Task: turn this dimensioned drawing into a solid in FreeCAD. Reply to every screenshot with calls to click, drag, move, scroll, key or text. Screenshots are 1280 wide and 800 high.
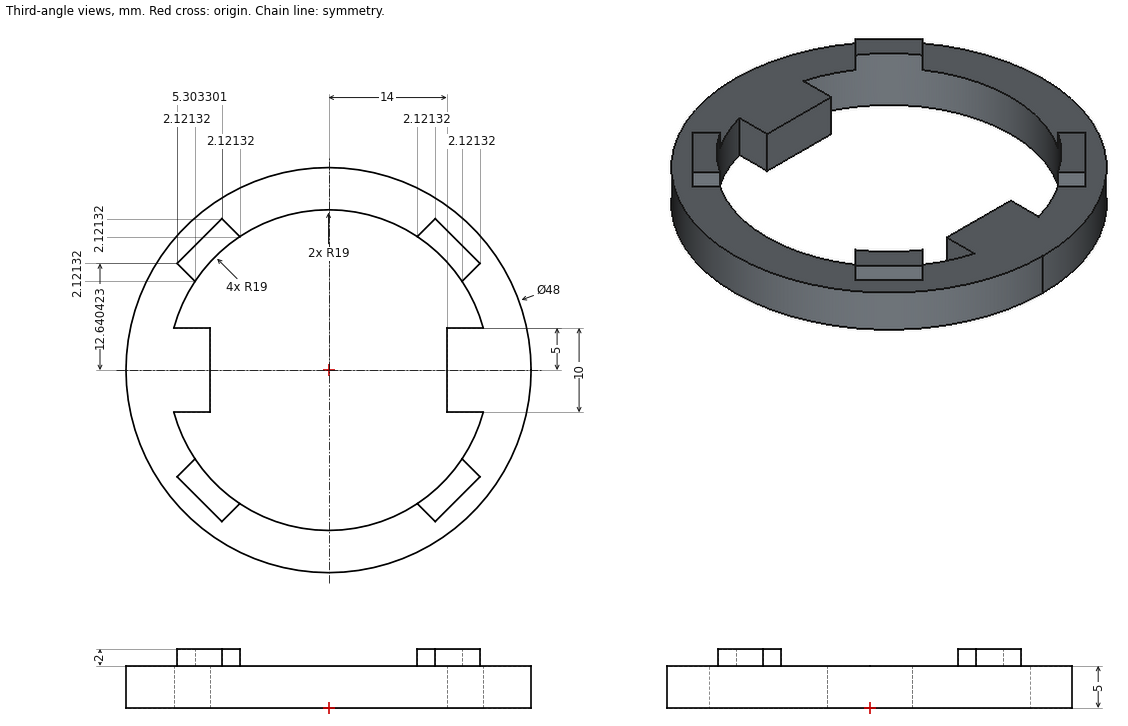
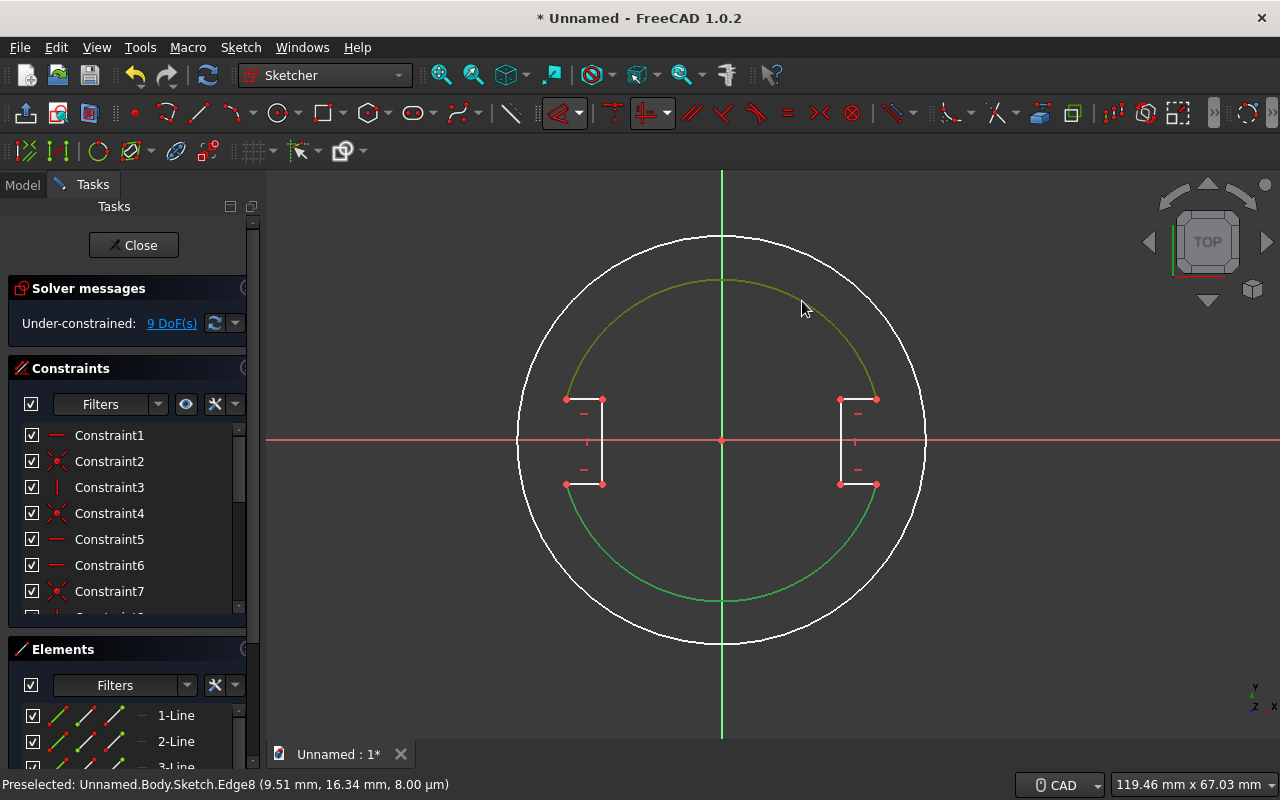
key(e)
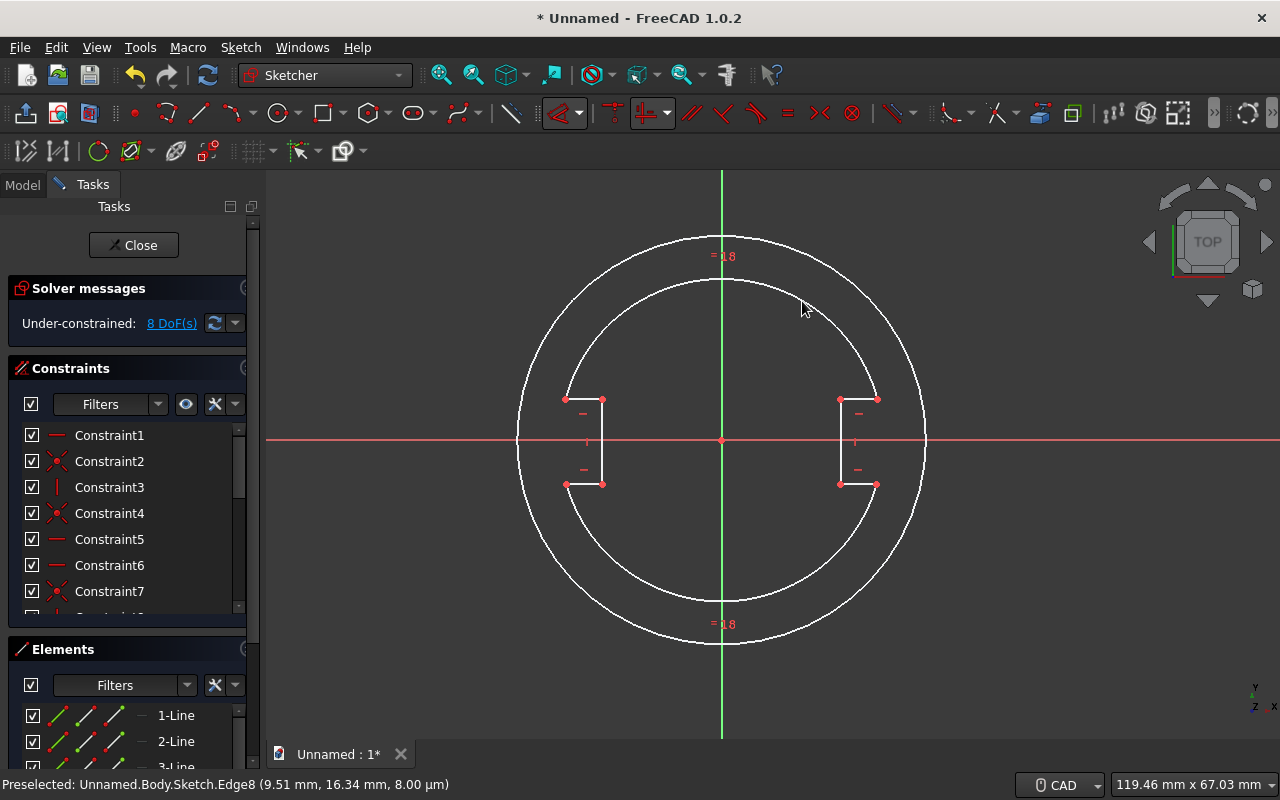
click(841, 484)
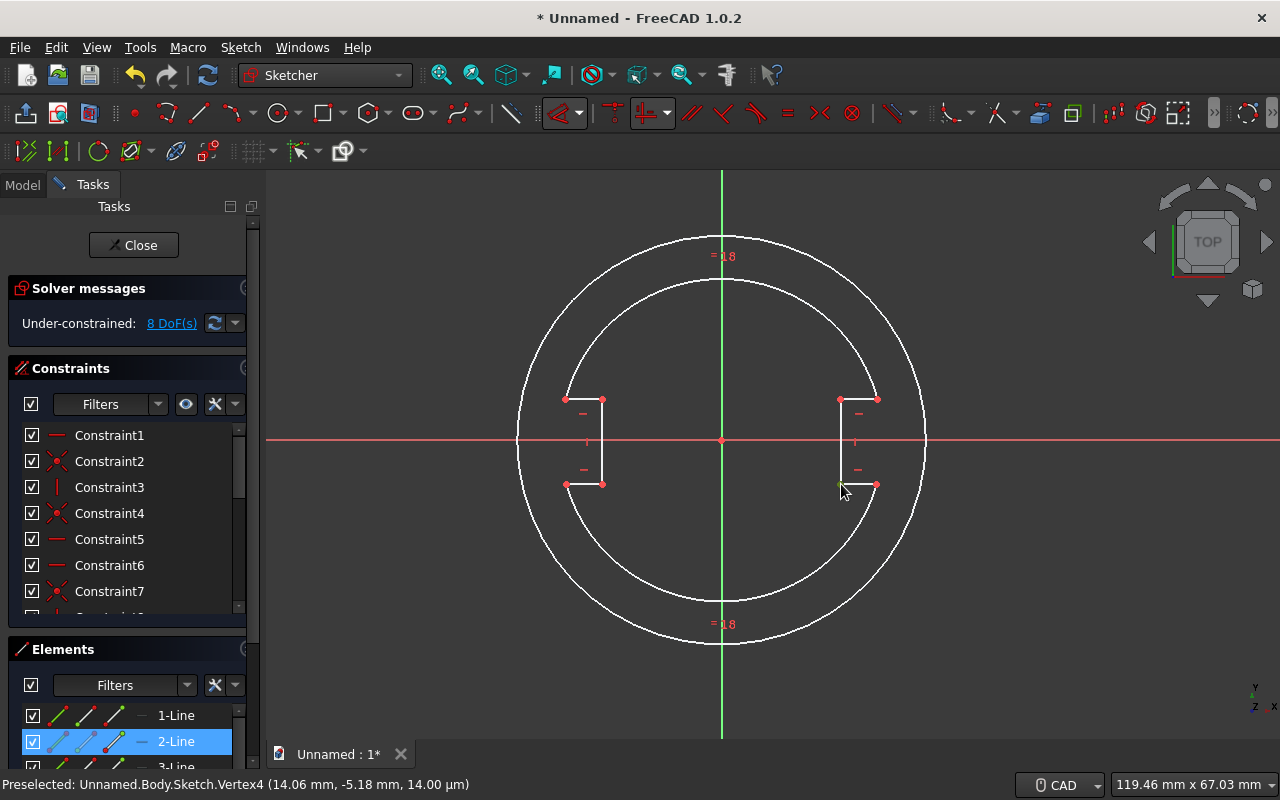
click(602, 484)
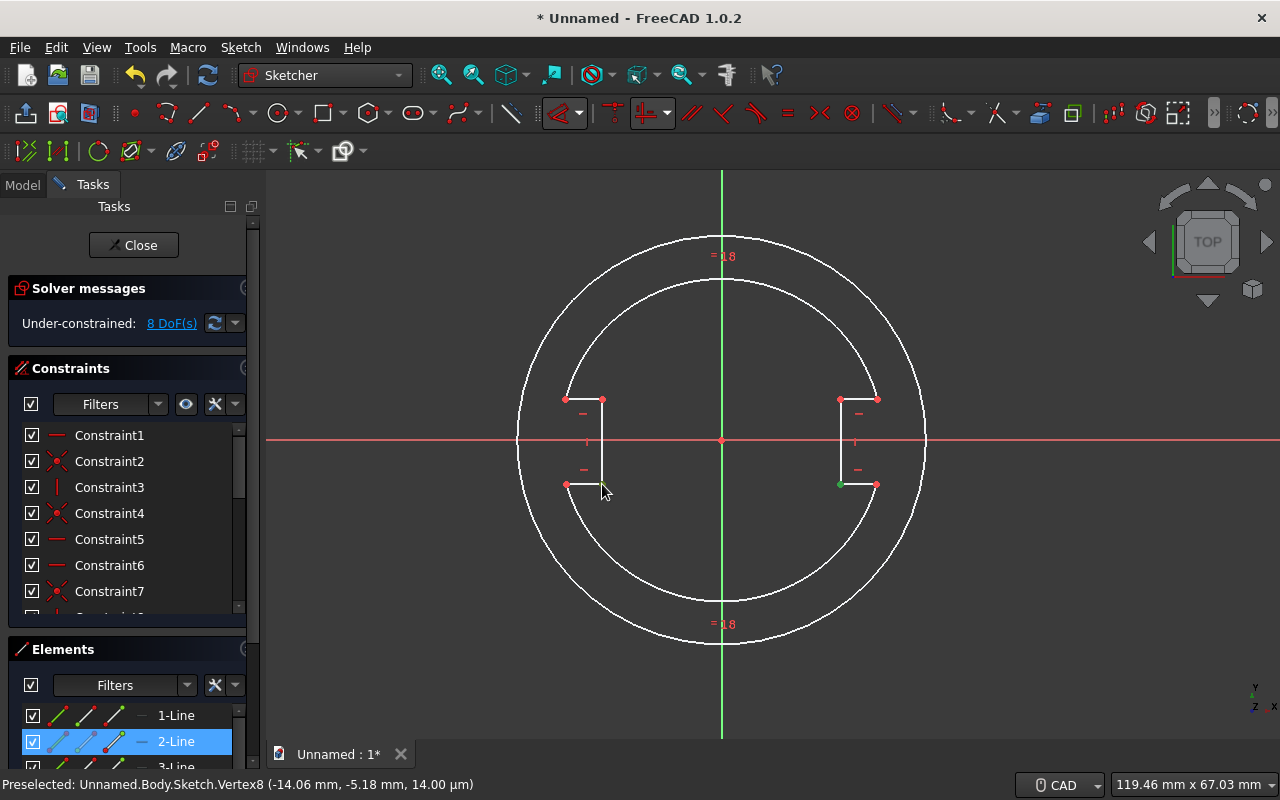
click(722, 564)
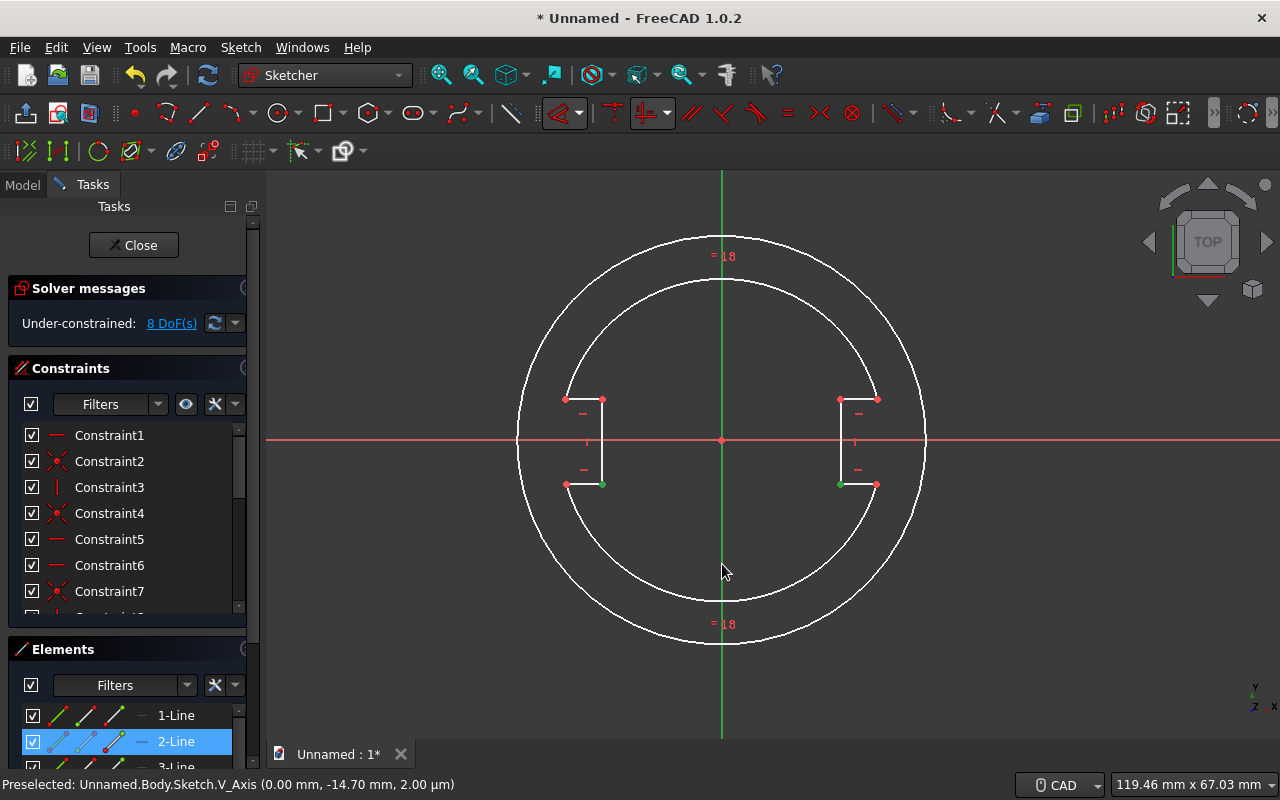
key(s)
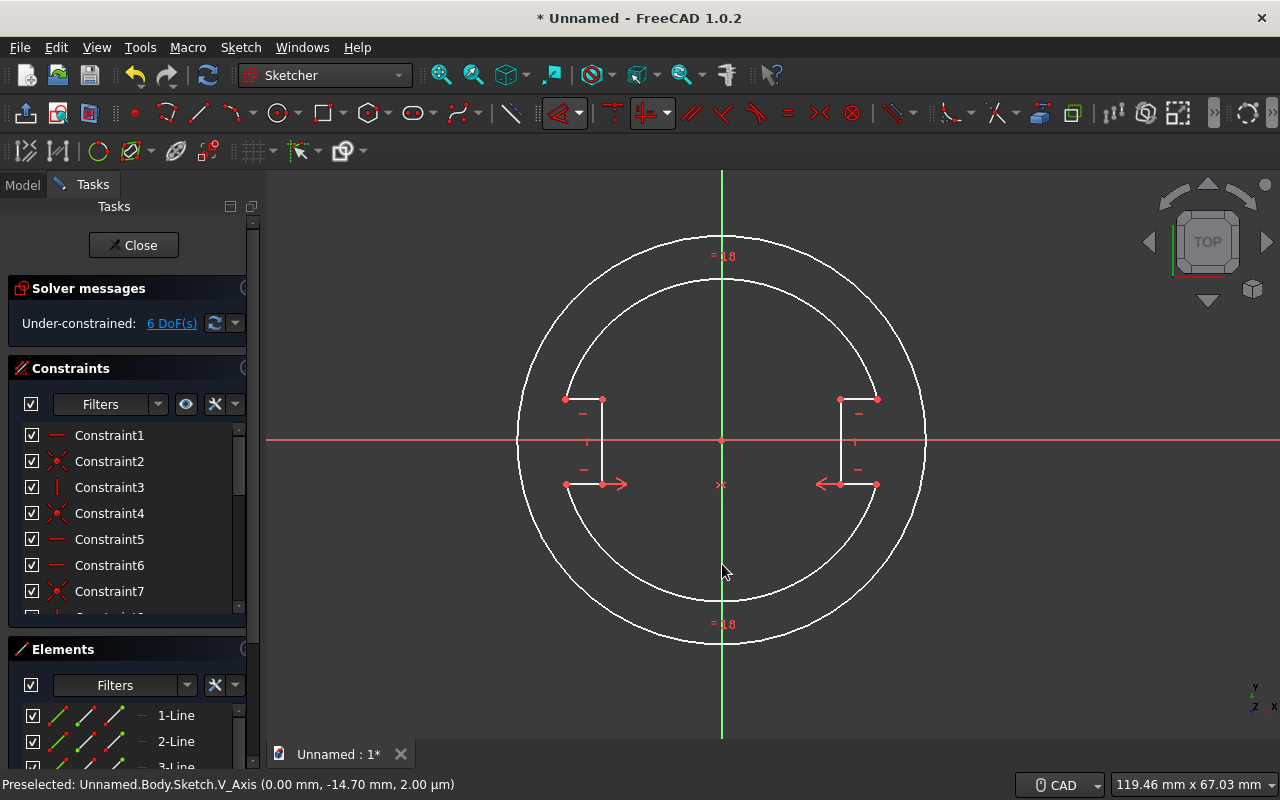
click(558, 114)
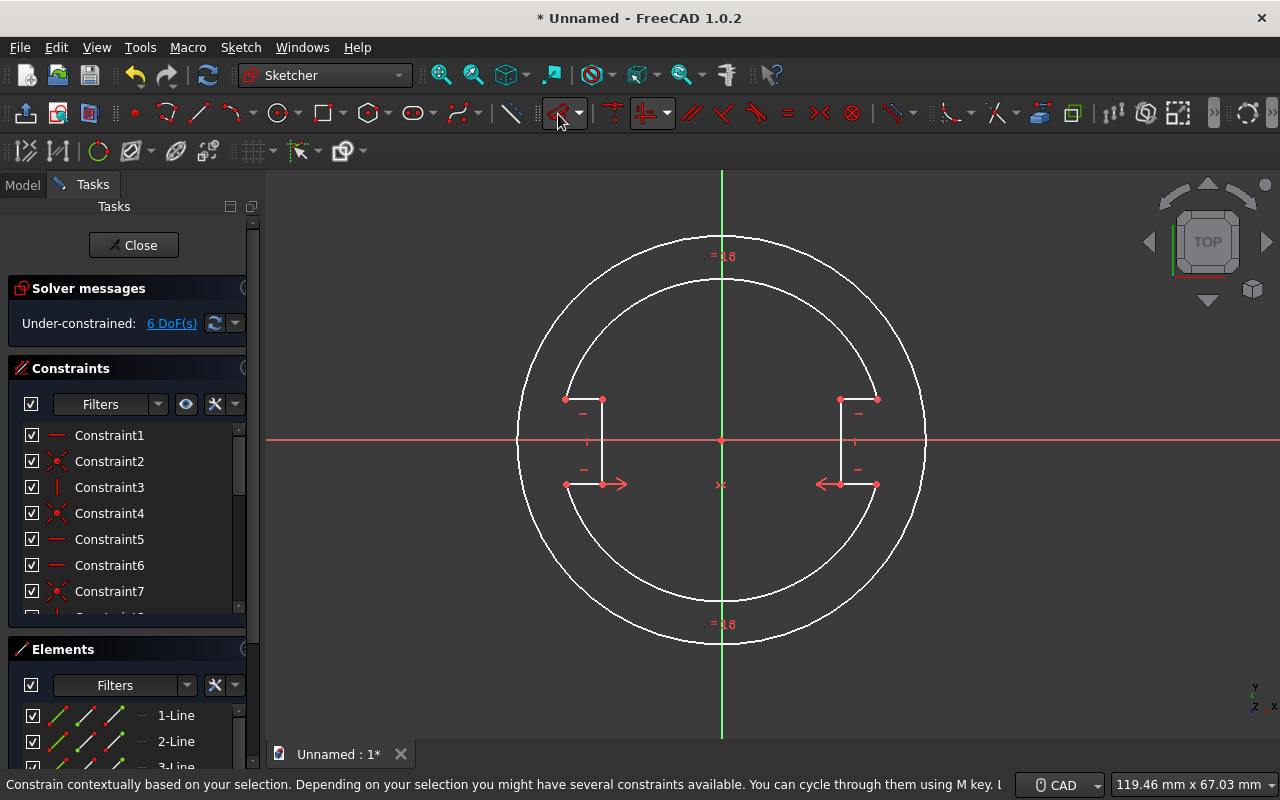
click(642, 580)
click(602, 650)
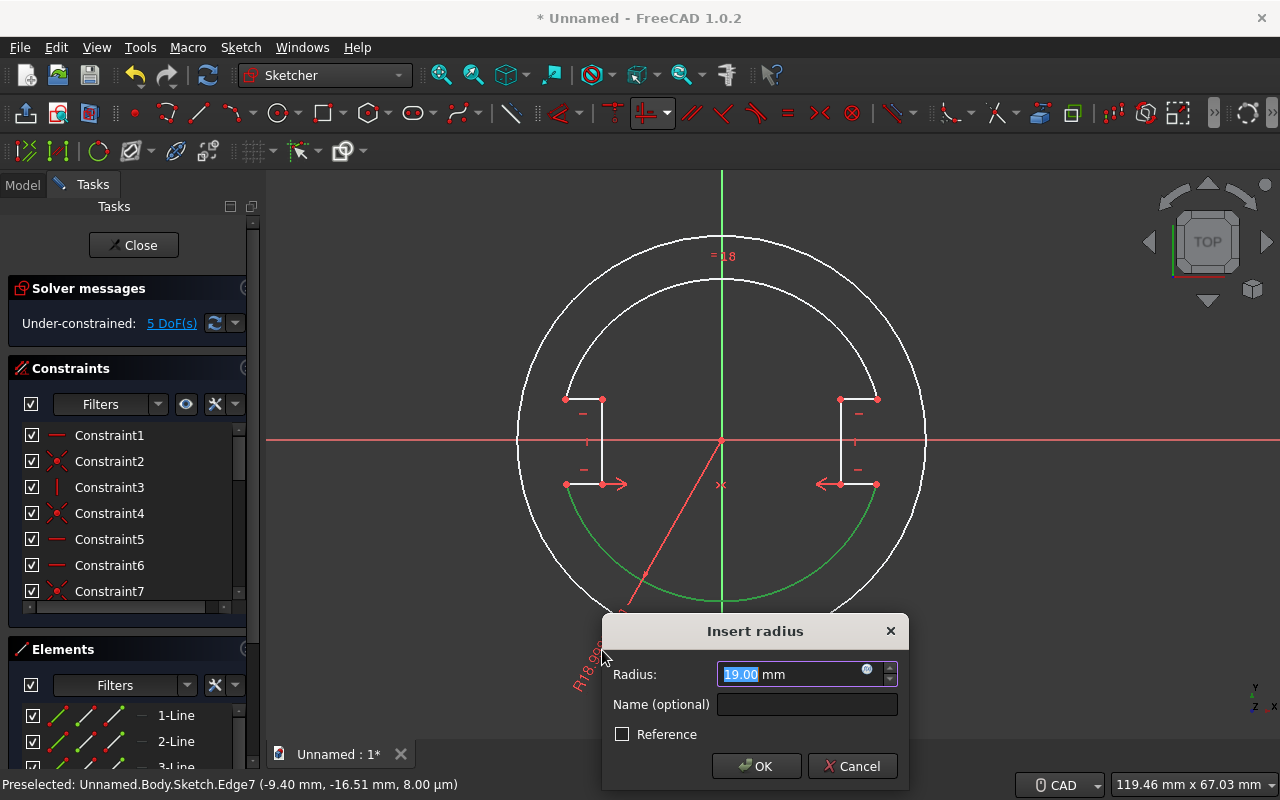
text(19)
key(Return)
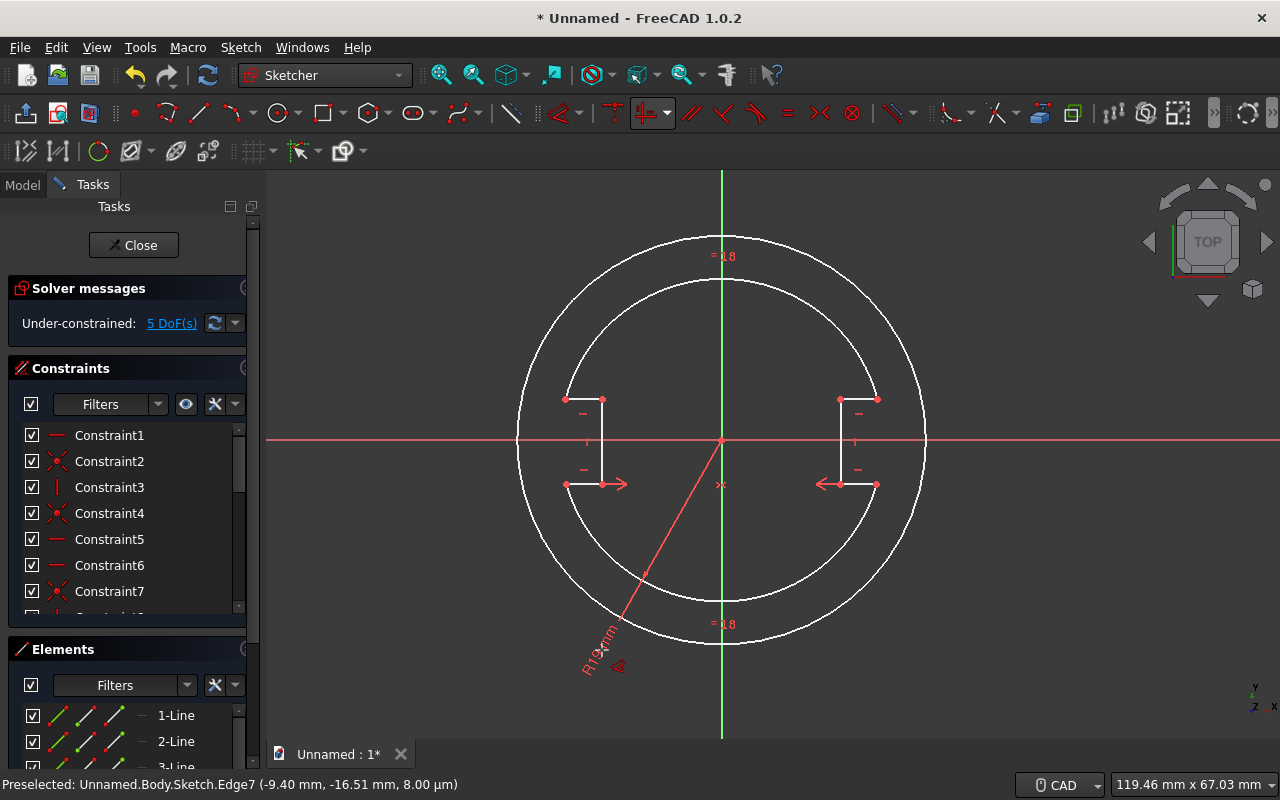
click(866, 295)
click(889, 272)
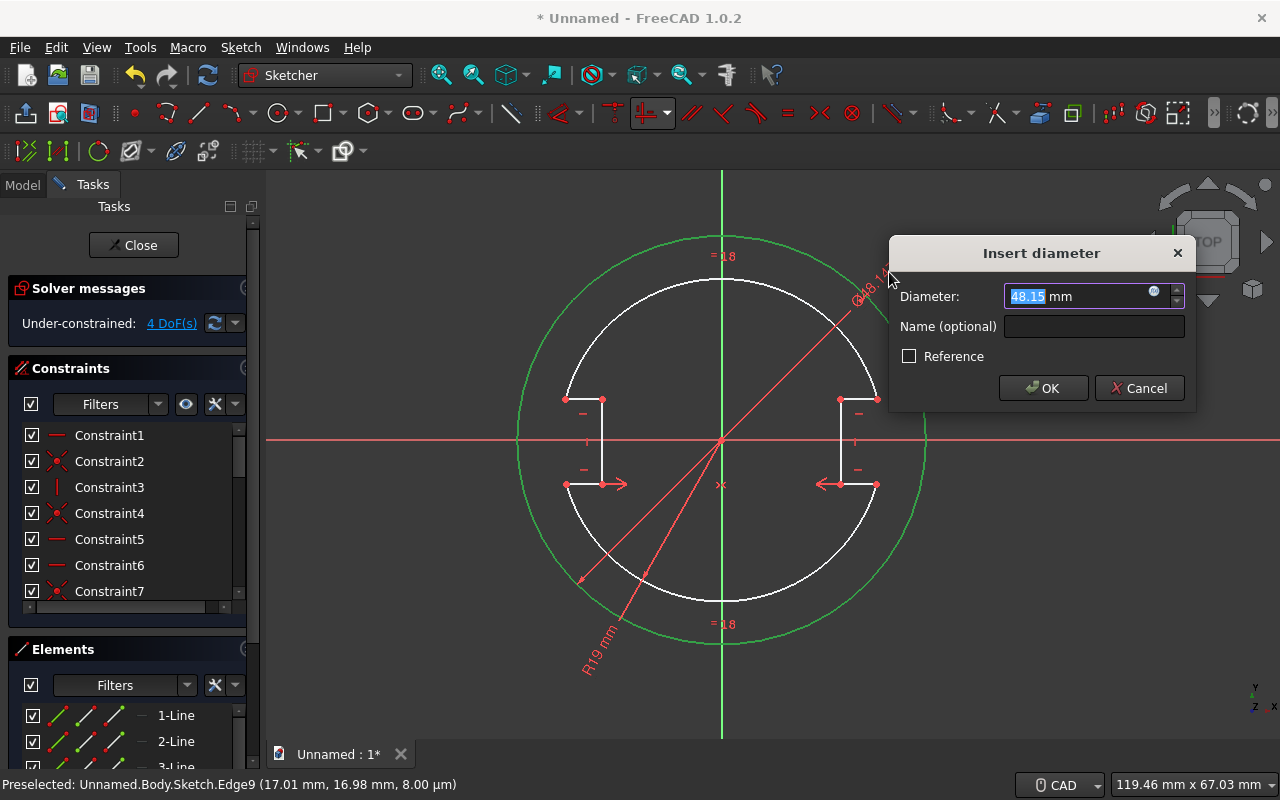
text(48)
key(Return)